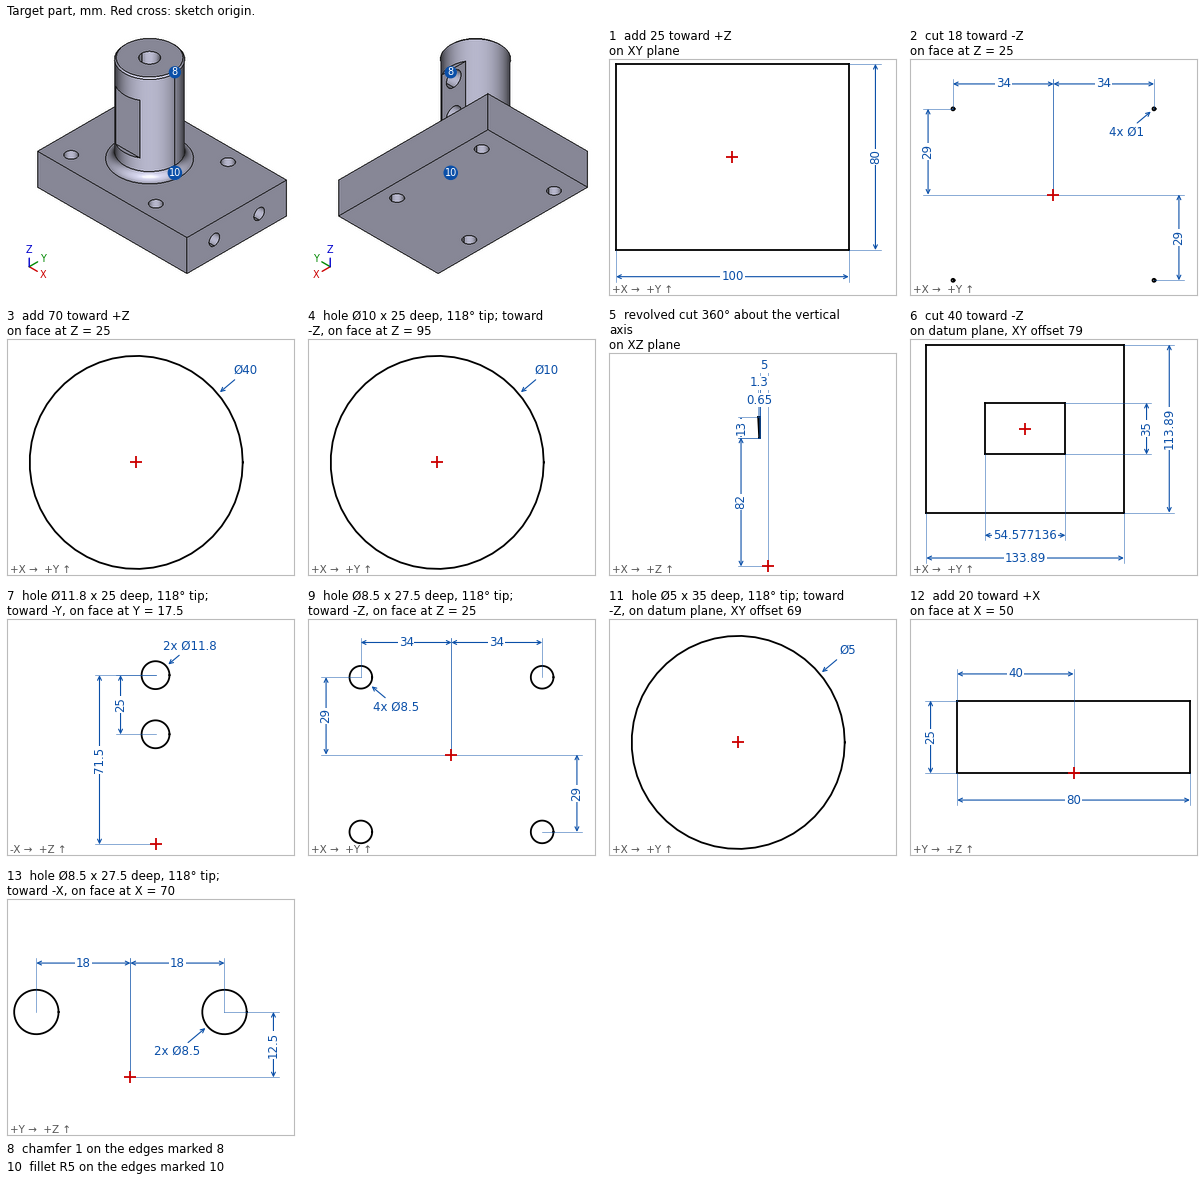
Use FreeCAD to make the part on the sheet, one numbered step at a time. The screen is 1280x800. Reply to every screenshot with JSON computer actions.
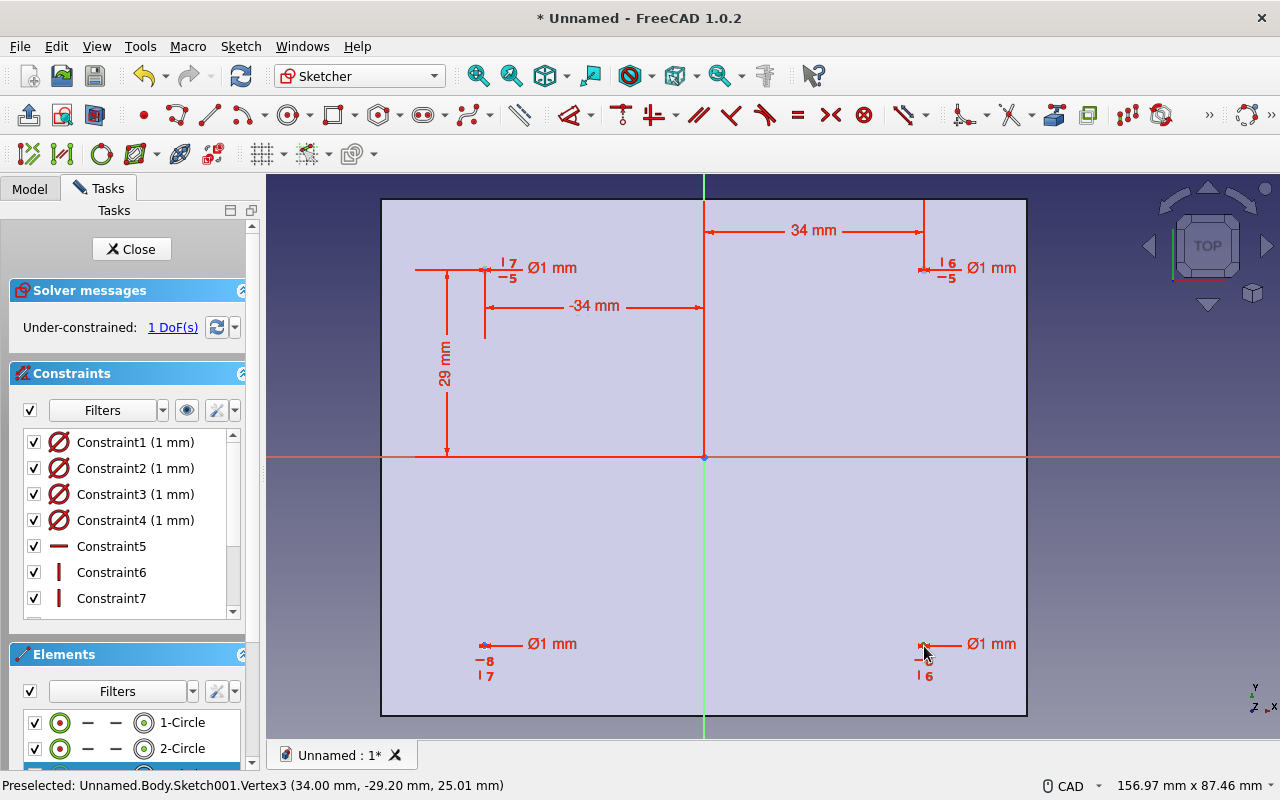
{"action": "key", "text": "i"}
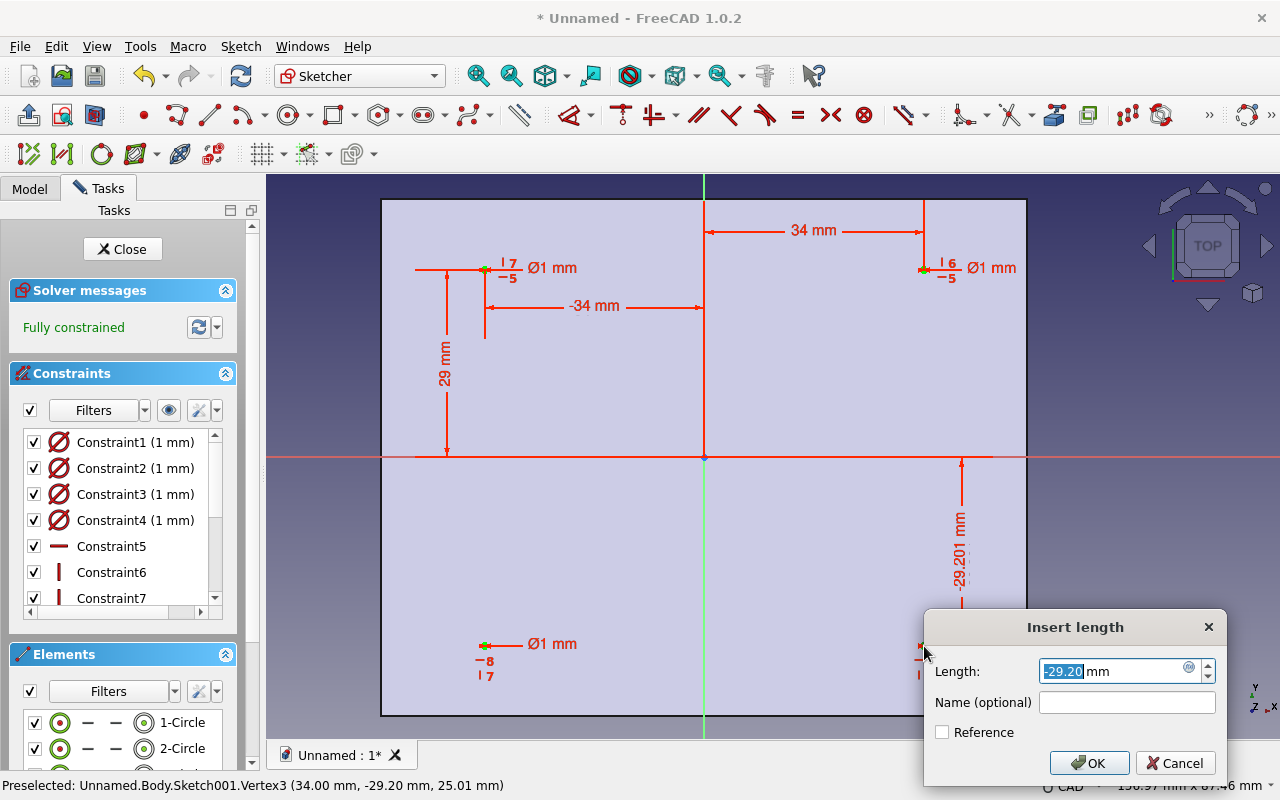
{"action": "type", "text": "-29"}
{"action": "key", "text": "Return"}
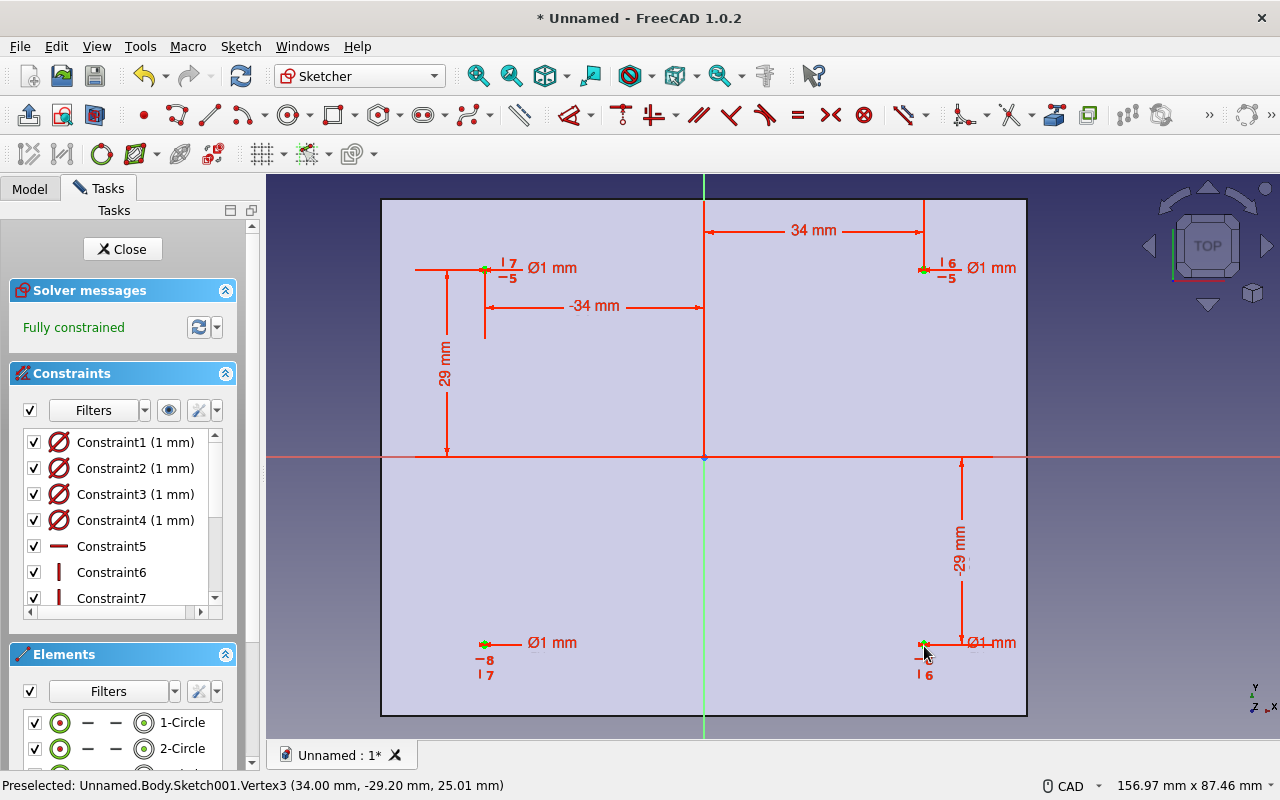
{"action": "left_click", "coordinate": [123, 249]}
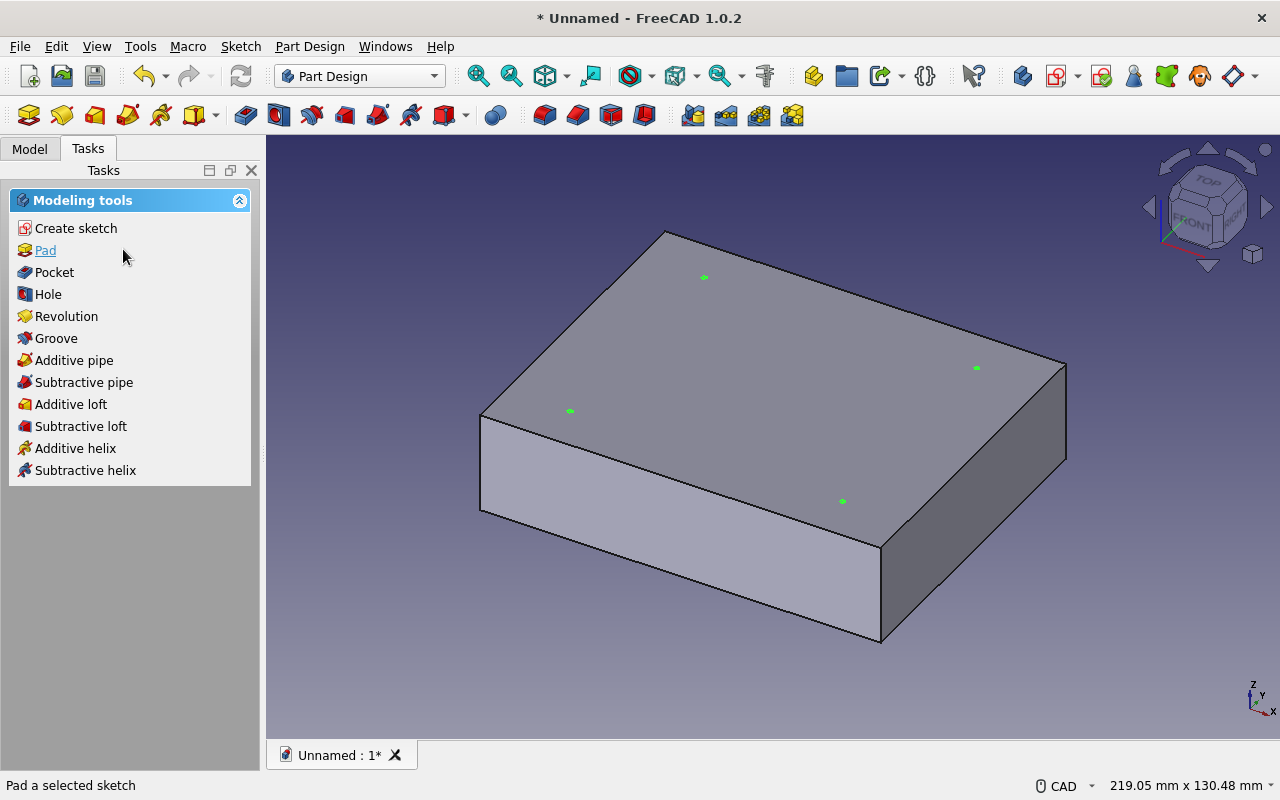
{"action": "left_click", "coordinate": [246, 116]}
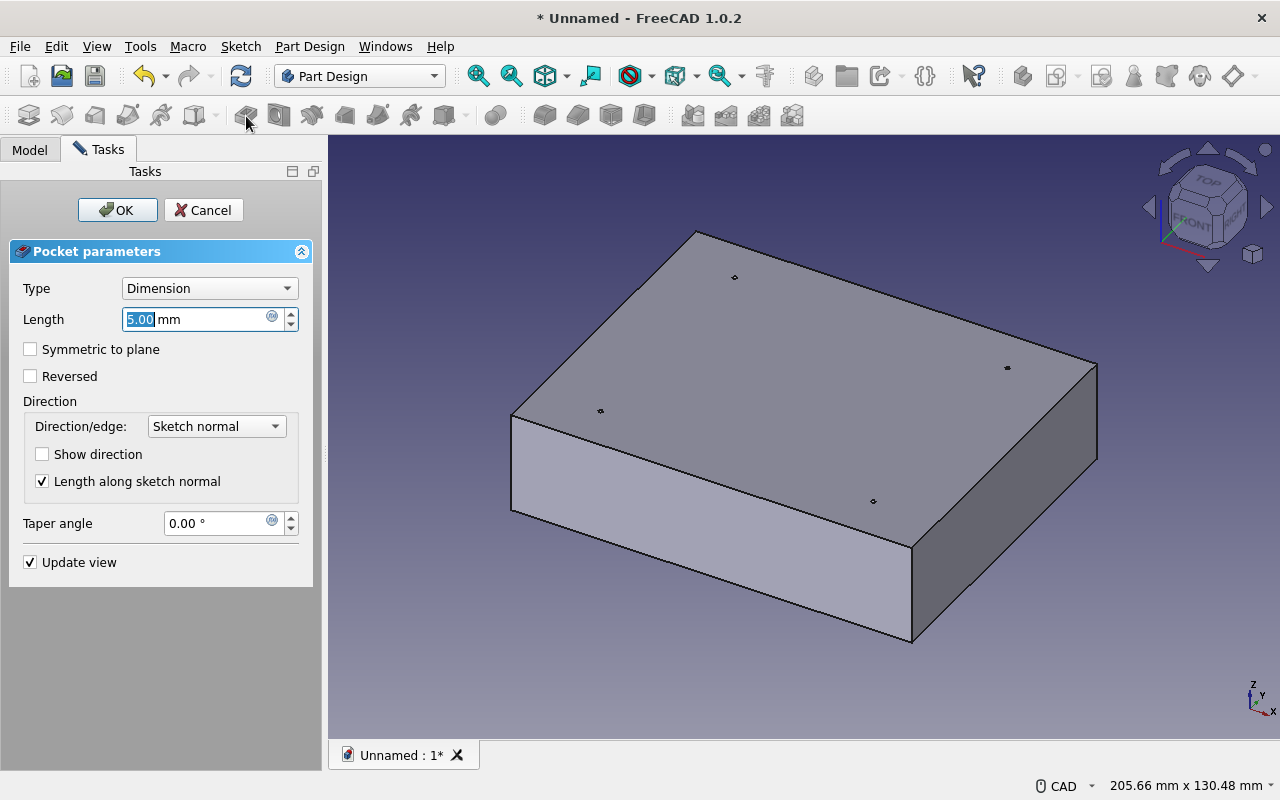
{"action": "type", "text": "18"}
{"action": "key", "text": "Tab"}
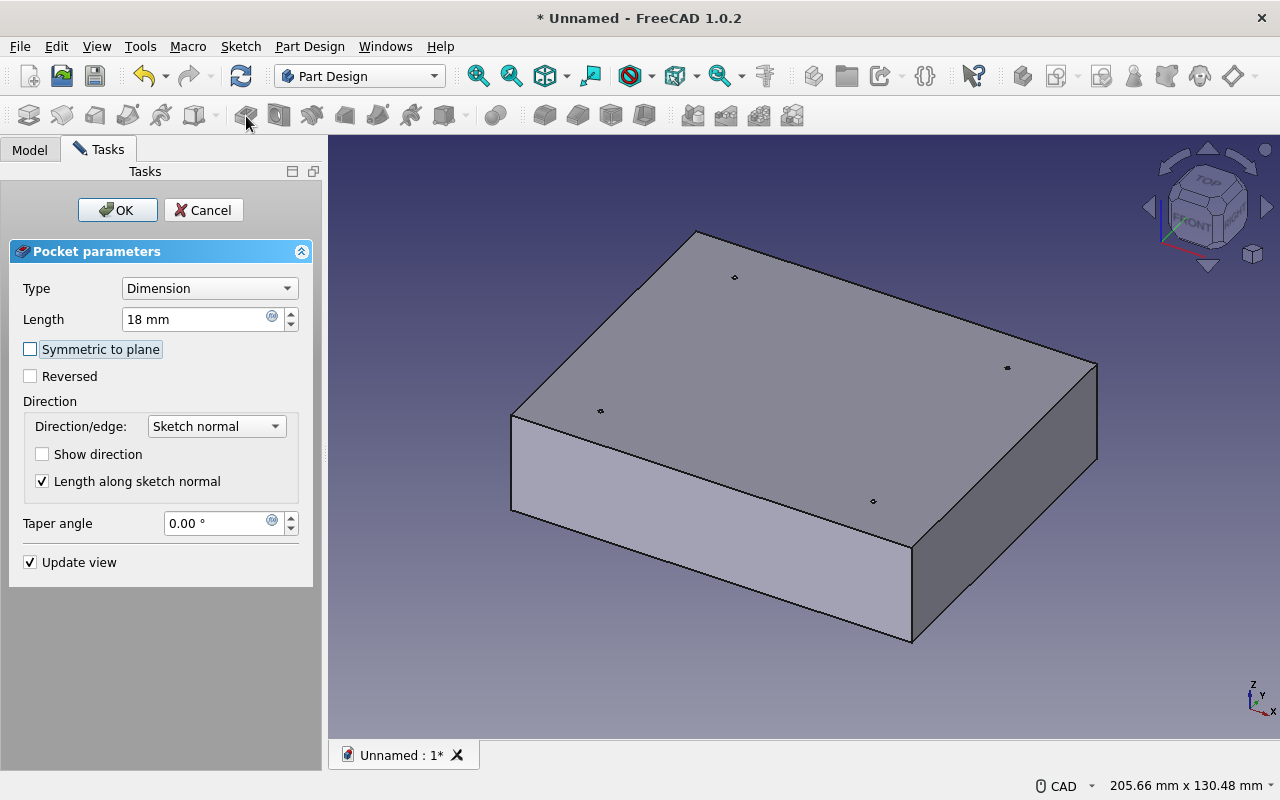
{"action": "left_click", "coordinate": [118, 210]}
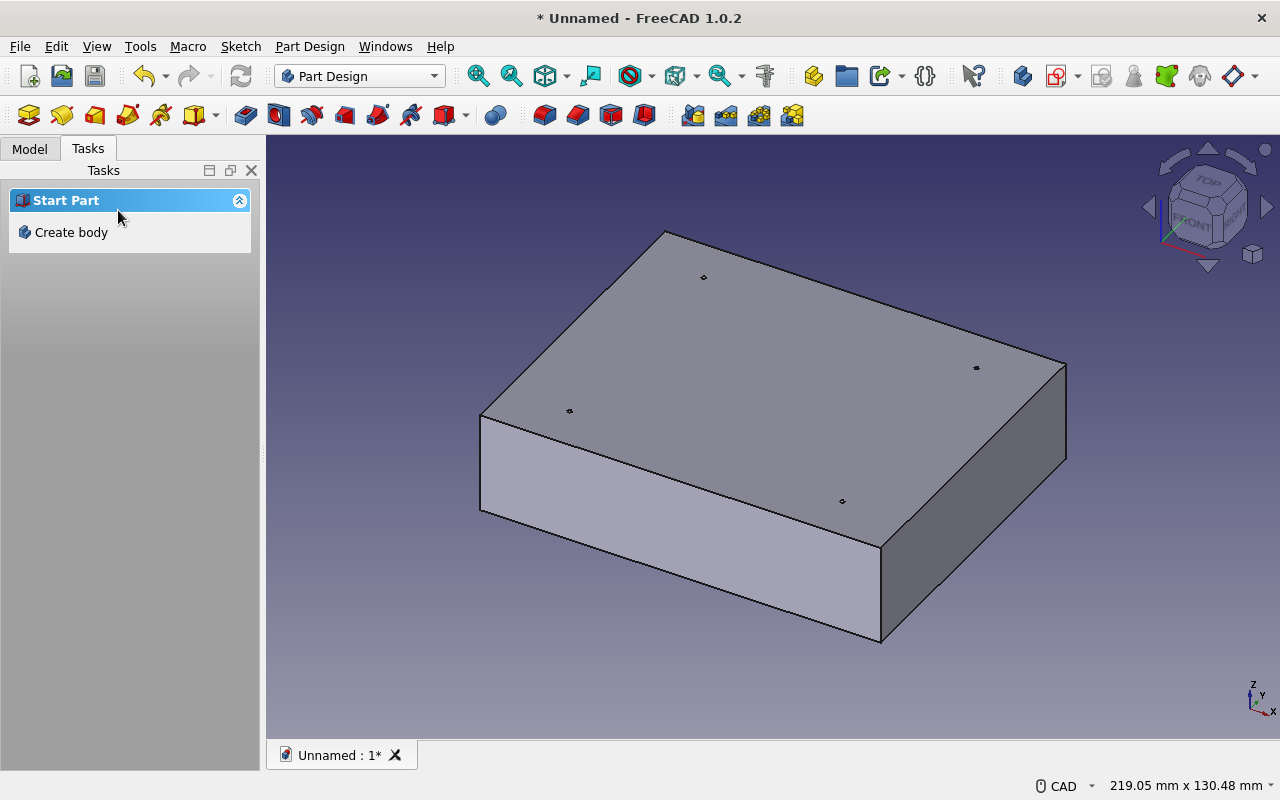
{"action": "left_click", "coordinate": [773, 389]}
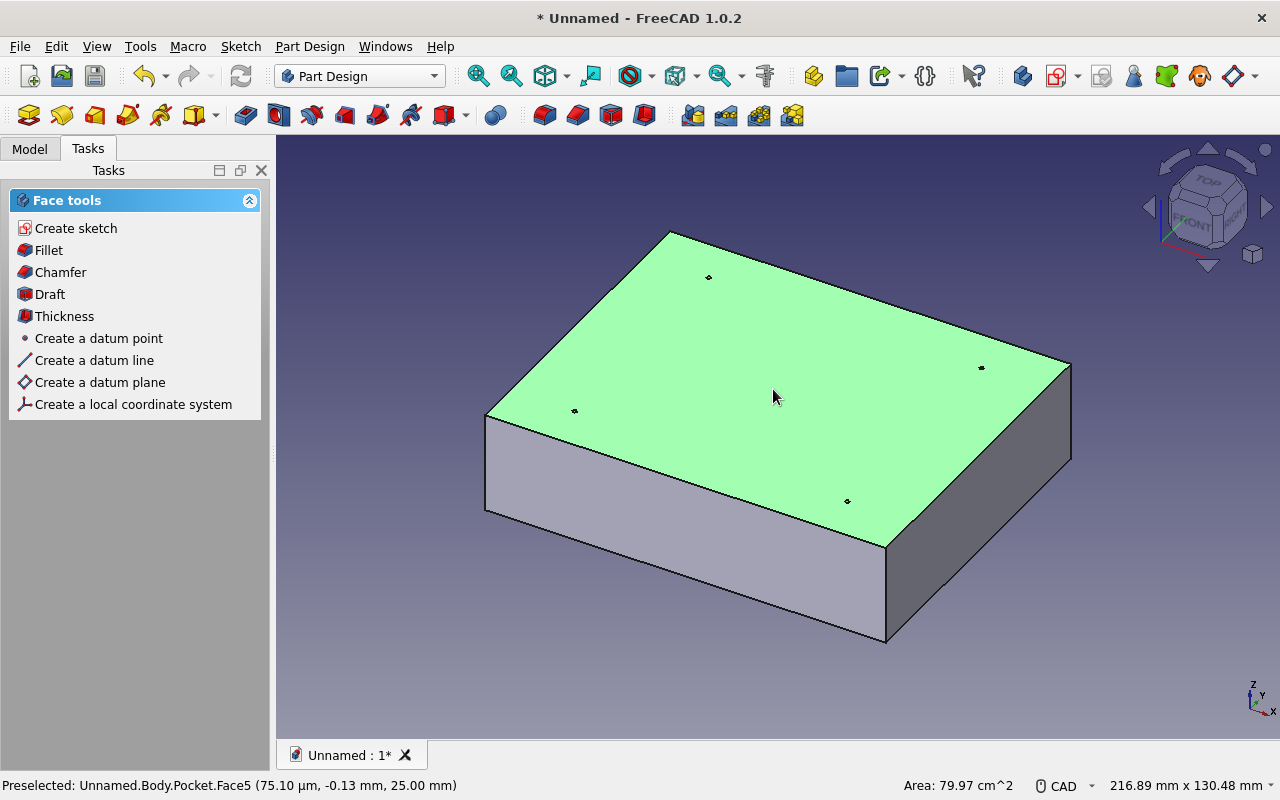
{"action": "left_click", "coordinate": [1056, 76]}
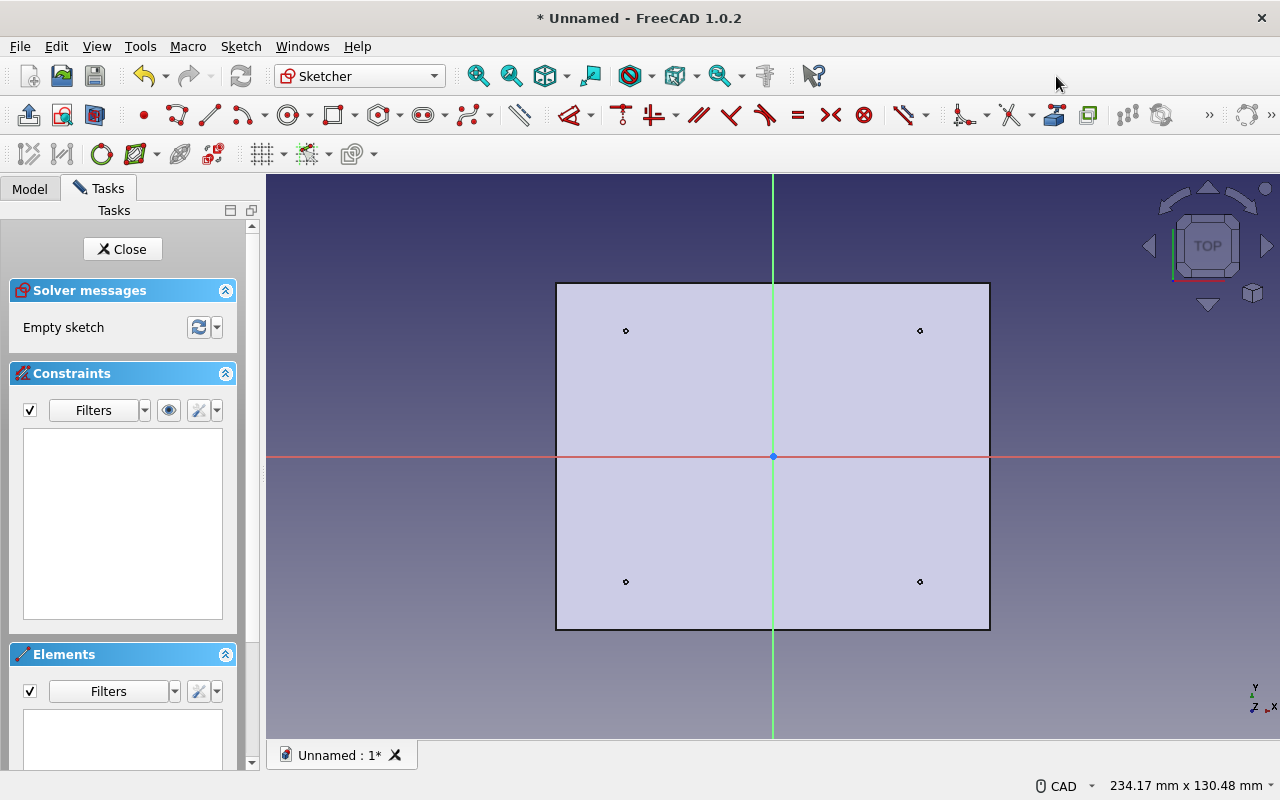
{"action": "scroll", "coordinate": [829, 456], "scroll_direction": "up", "scroll_amount": 4}